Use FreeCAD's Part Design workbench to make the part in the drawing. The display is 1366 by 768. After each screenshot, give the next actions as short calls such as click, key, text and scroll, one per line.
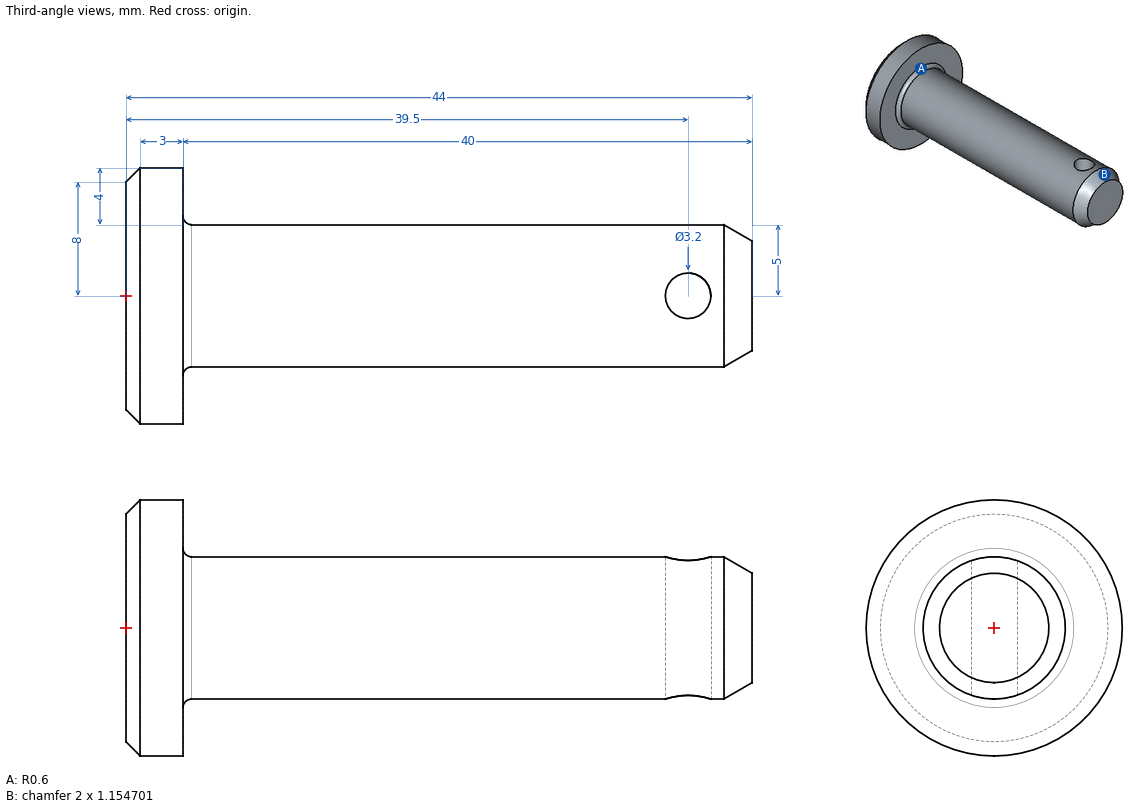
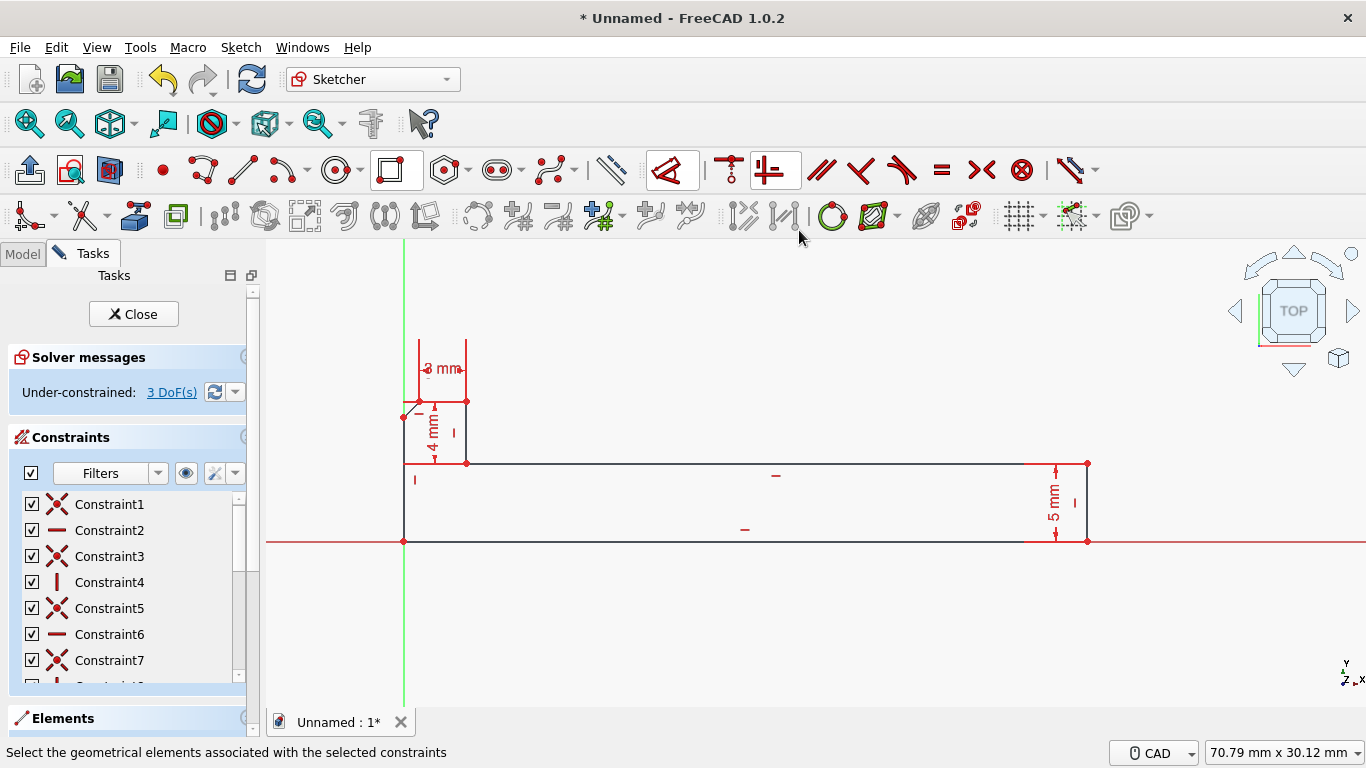
click(404, 455)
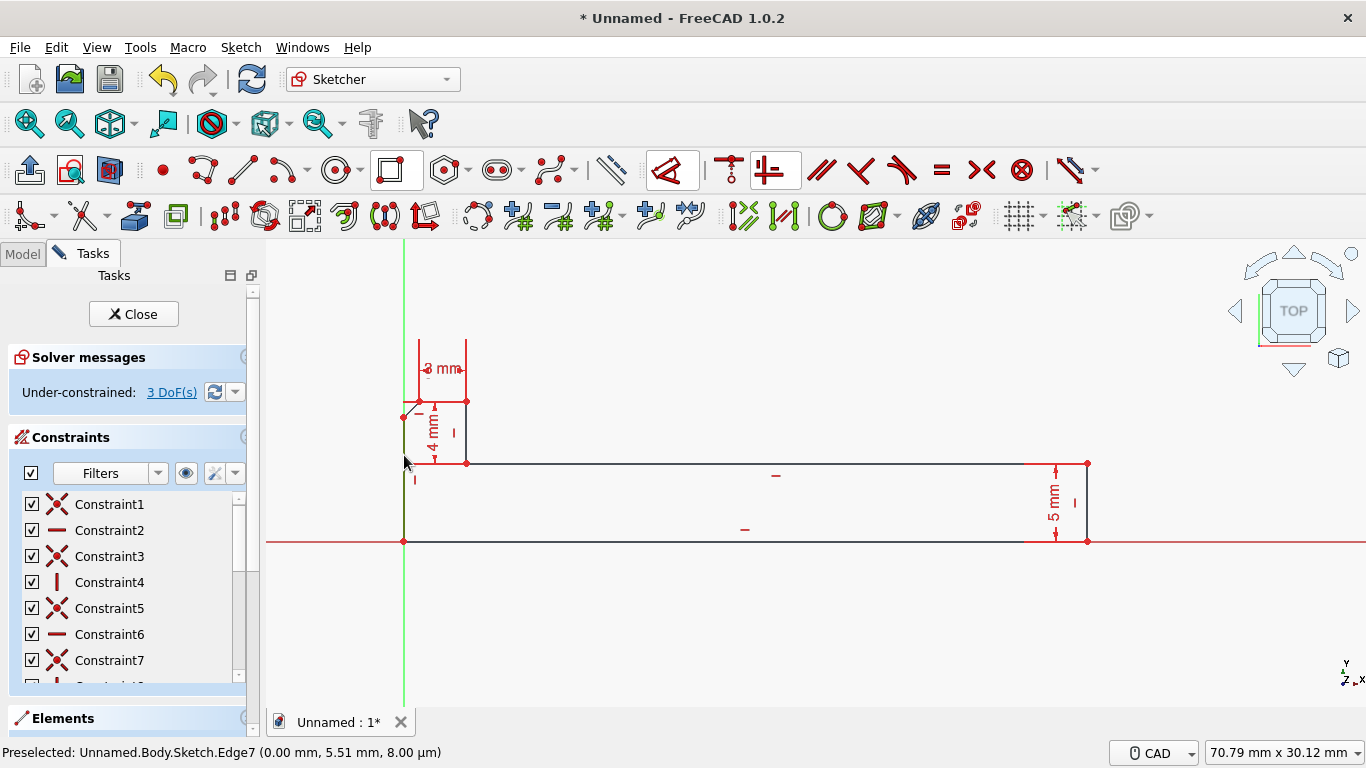
click(694, 170)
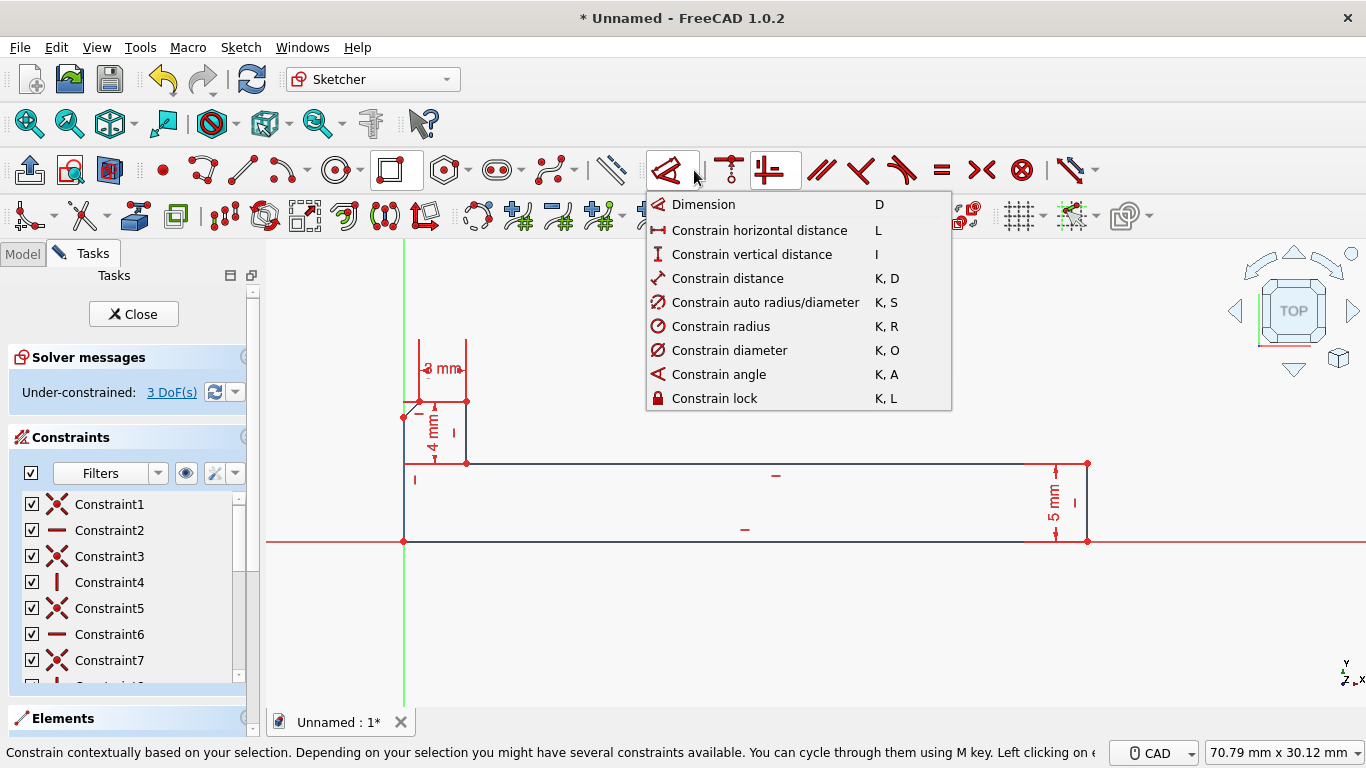
click(799, 254)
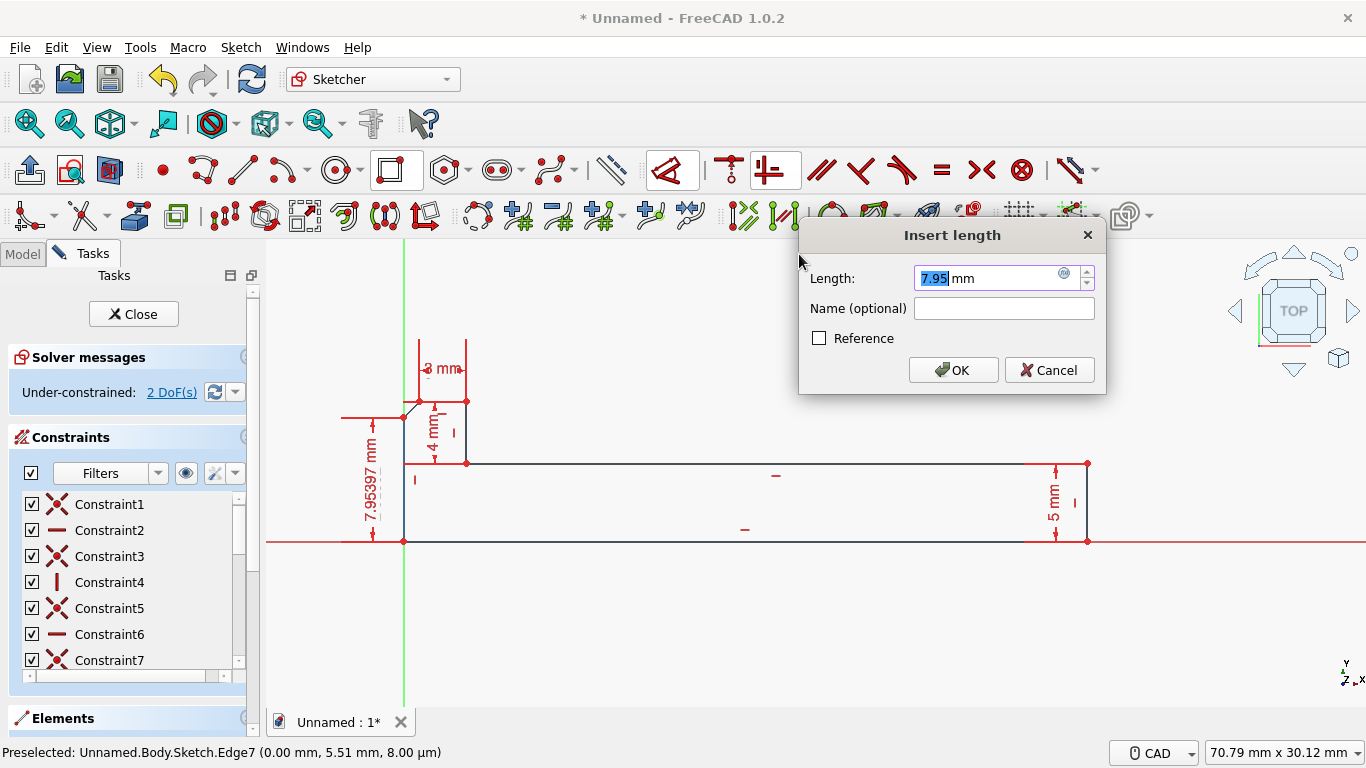
text(8)
key(Return)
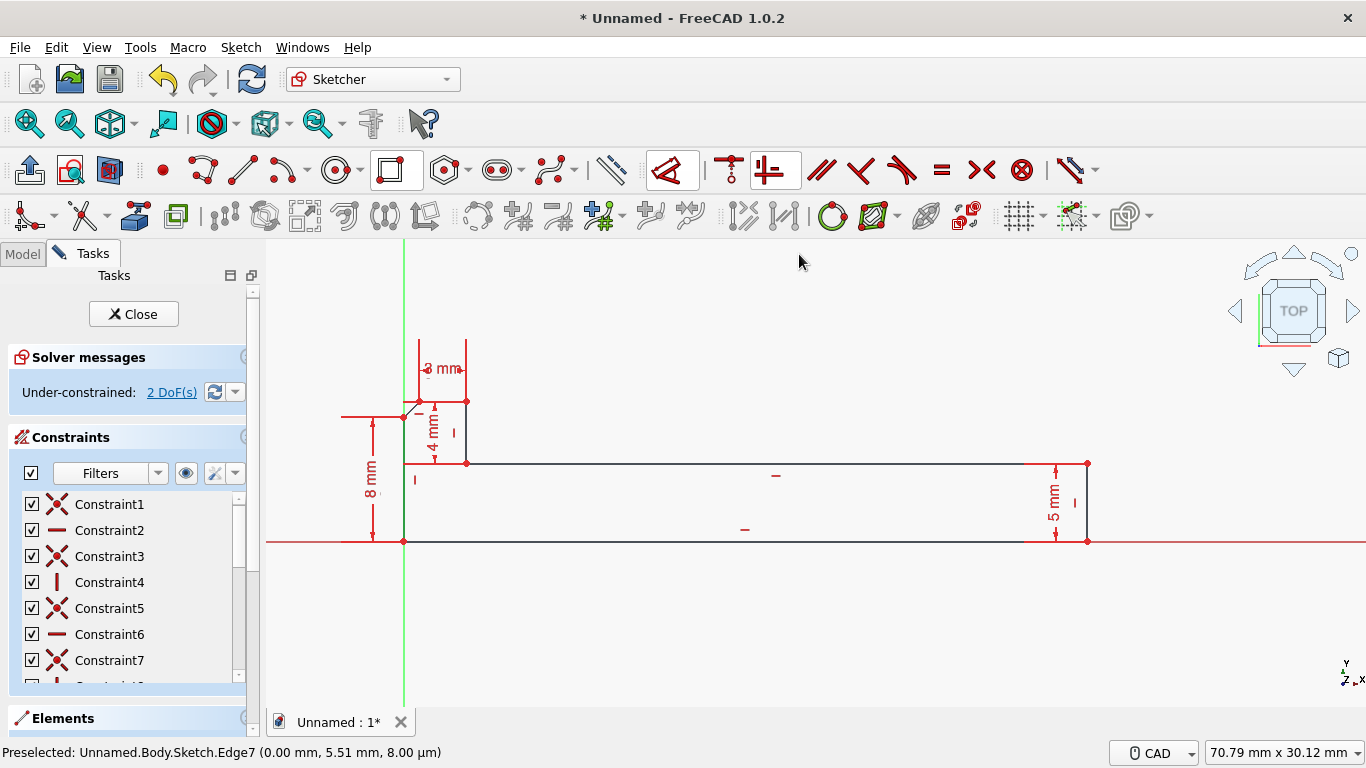
click(609, 542)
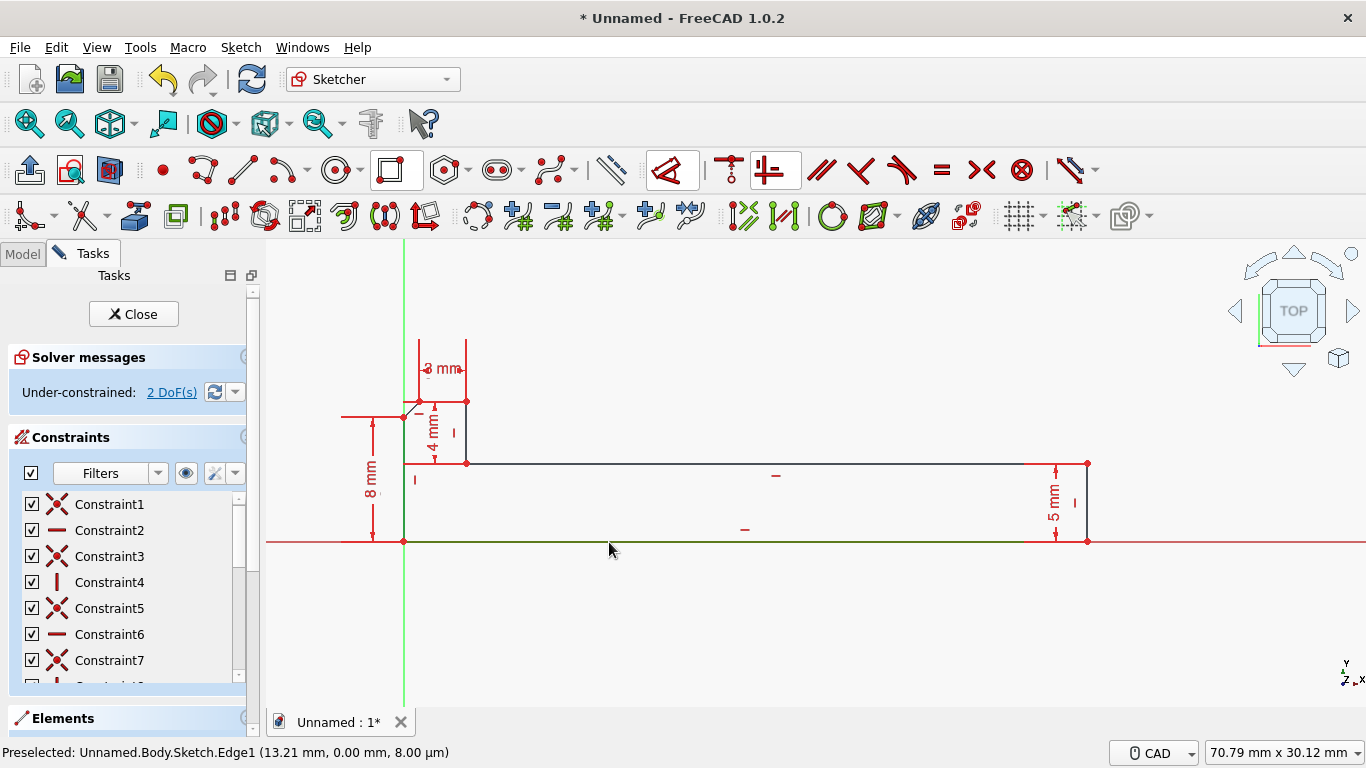
key(l)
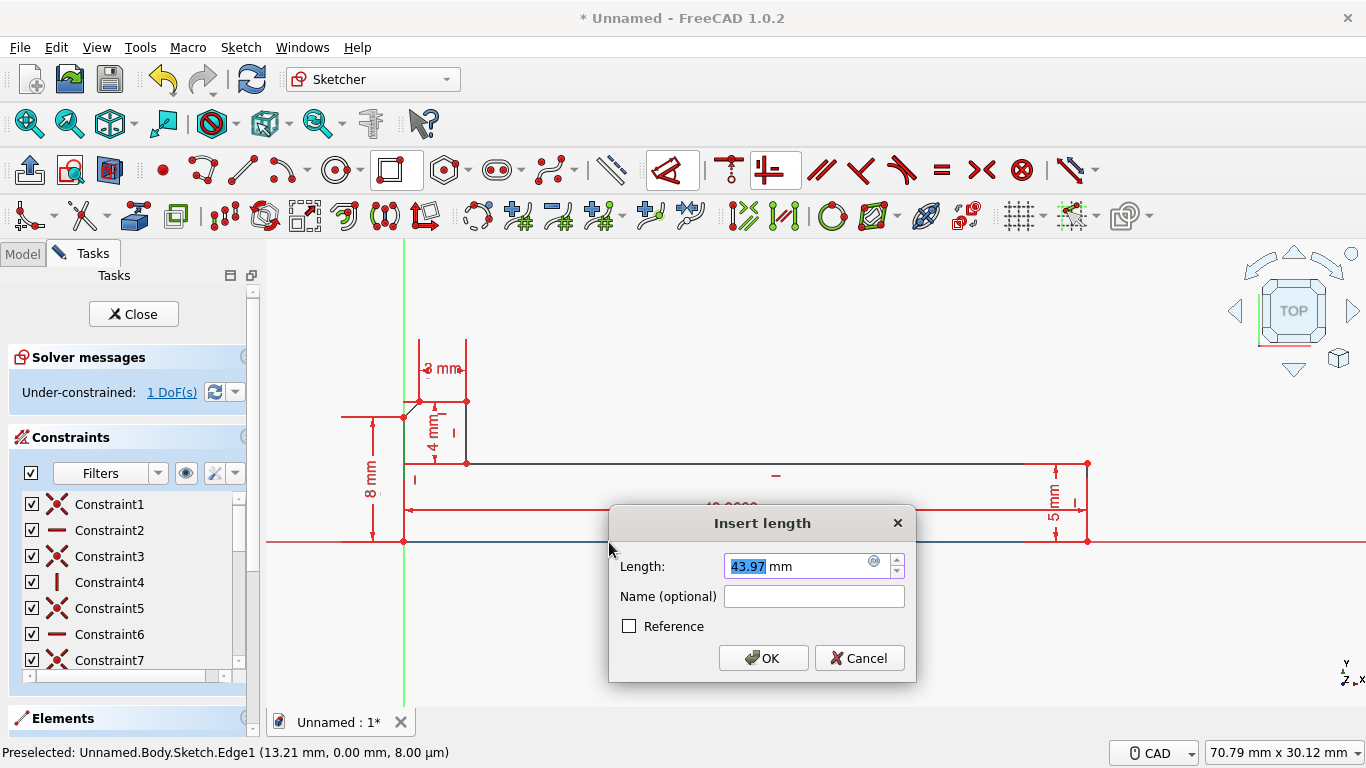
text(44)
key(Return)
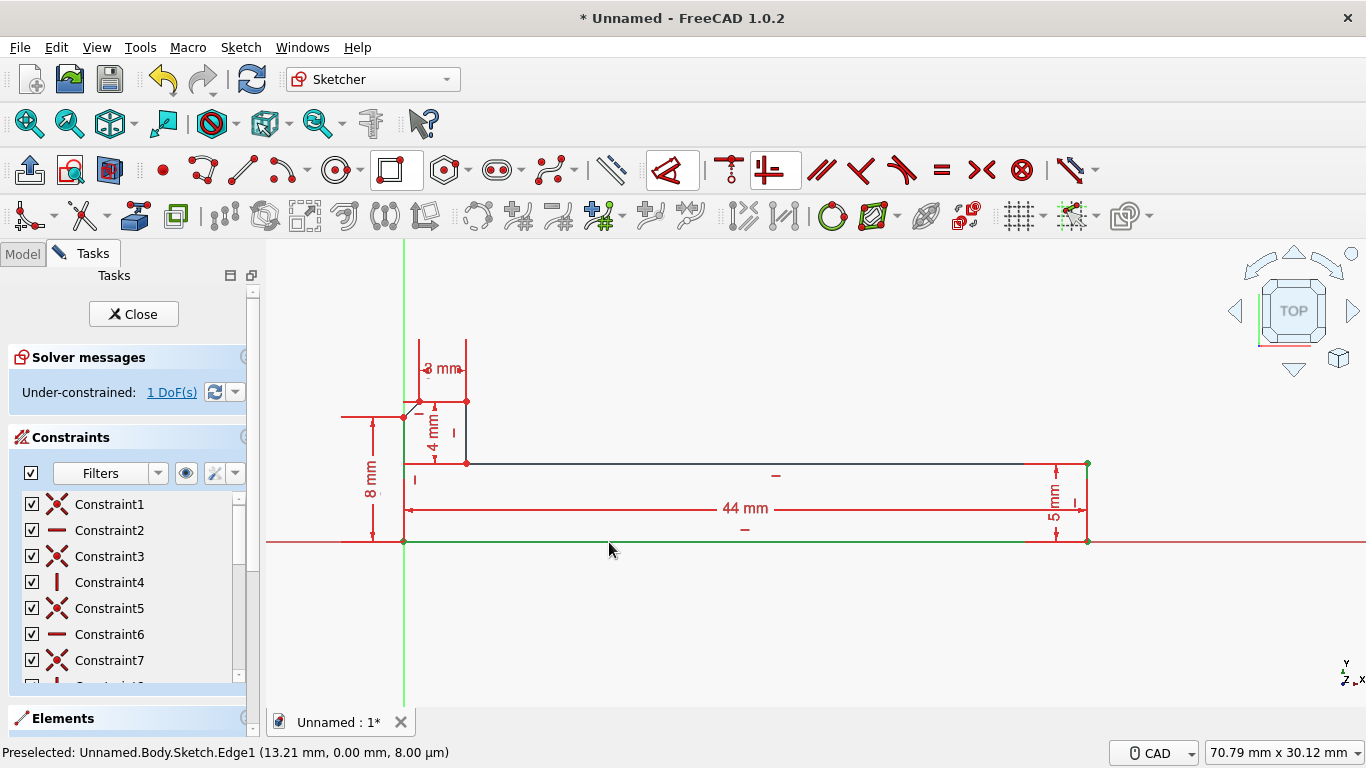
click(901, 464)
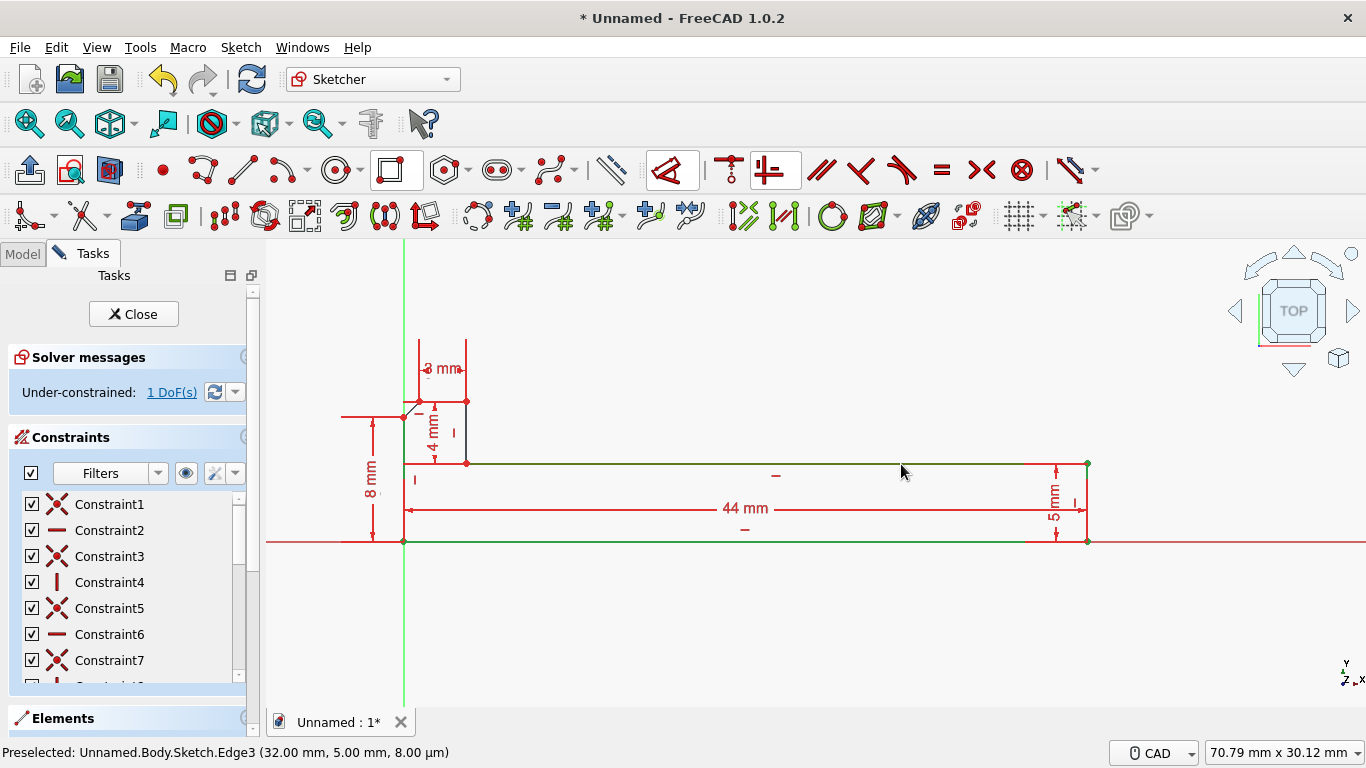
click(694, 170)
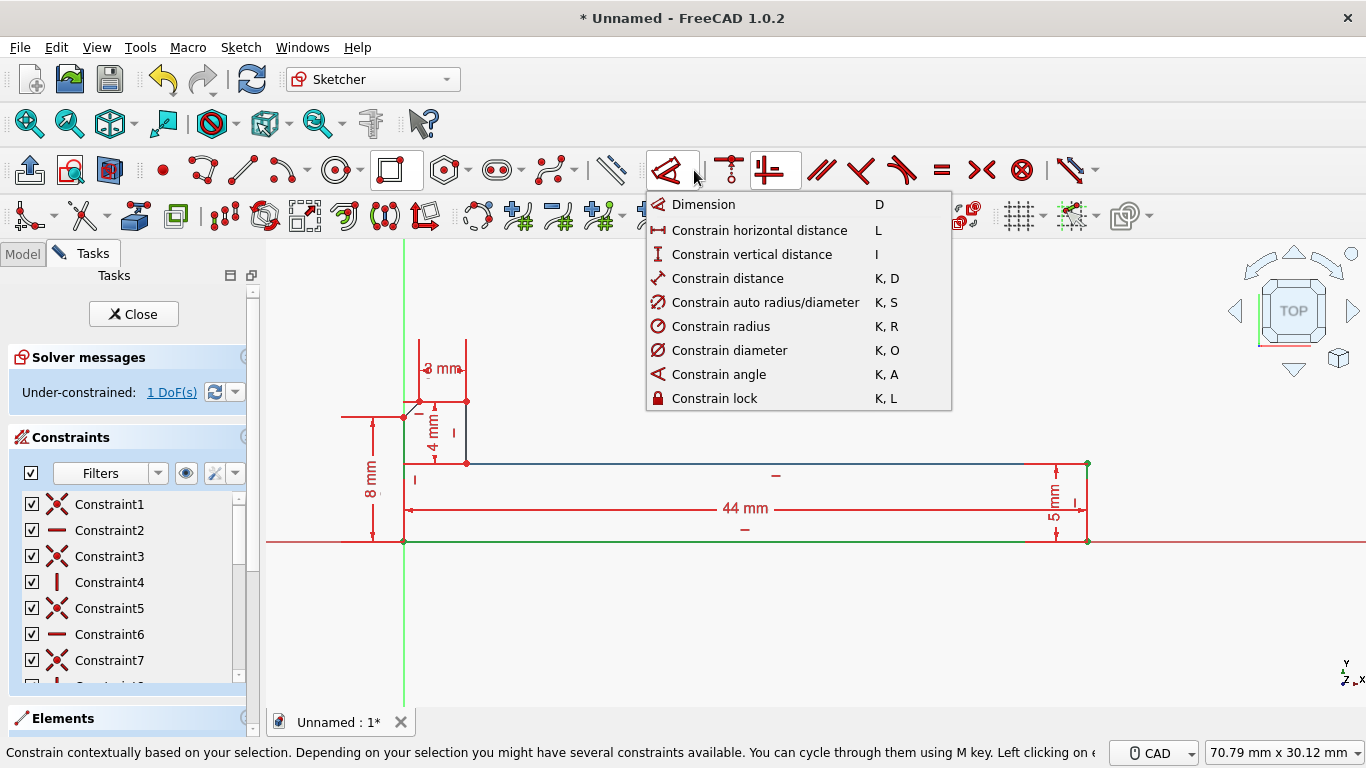
click(799, 230)